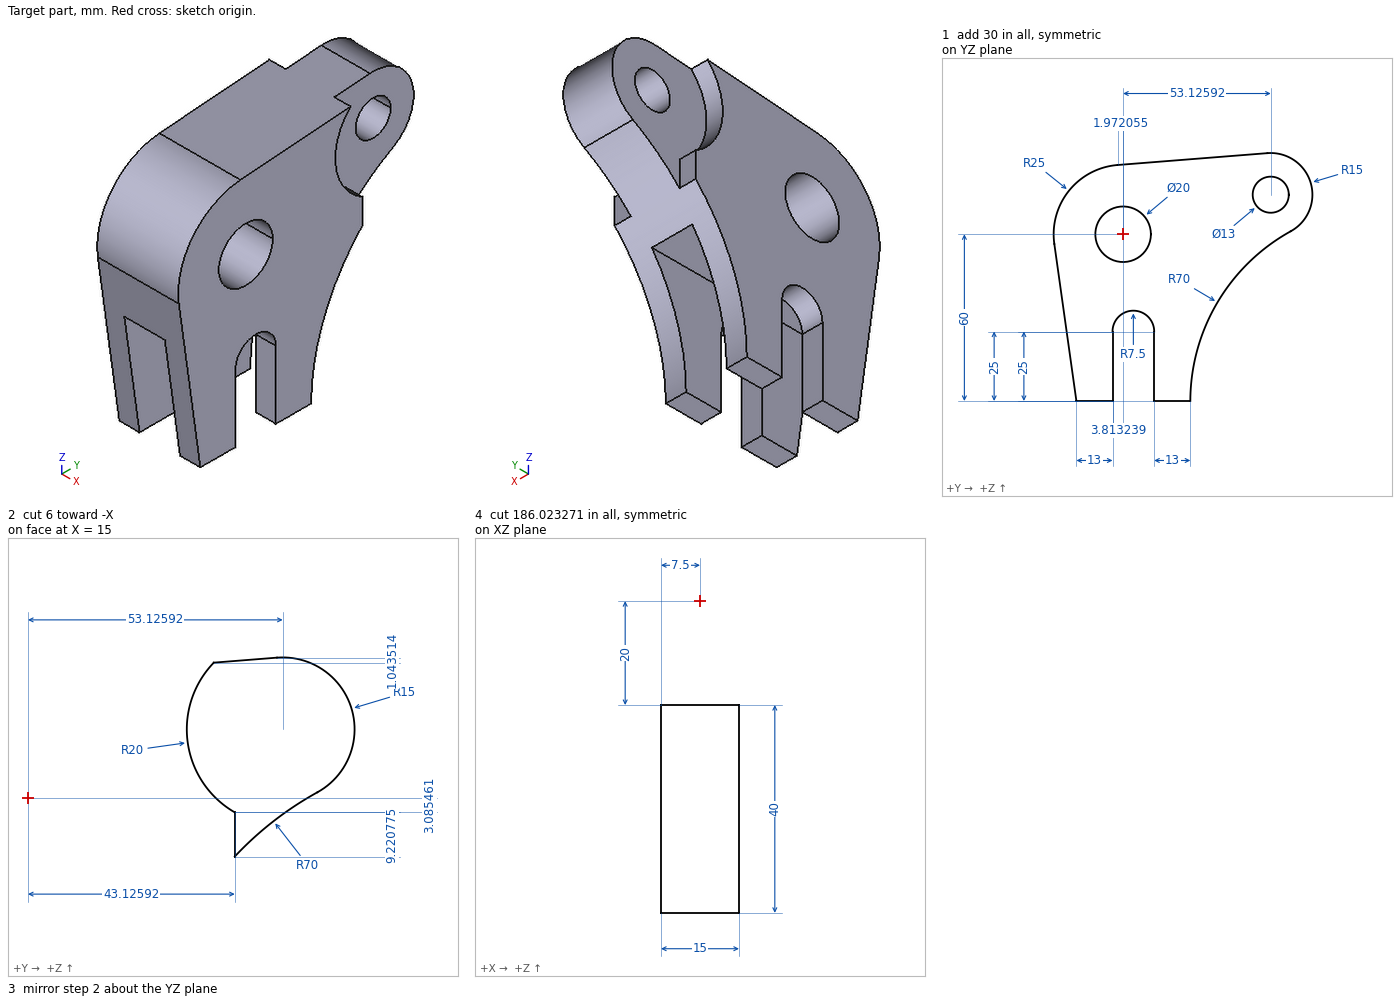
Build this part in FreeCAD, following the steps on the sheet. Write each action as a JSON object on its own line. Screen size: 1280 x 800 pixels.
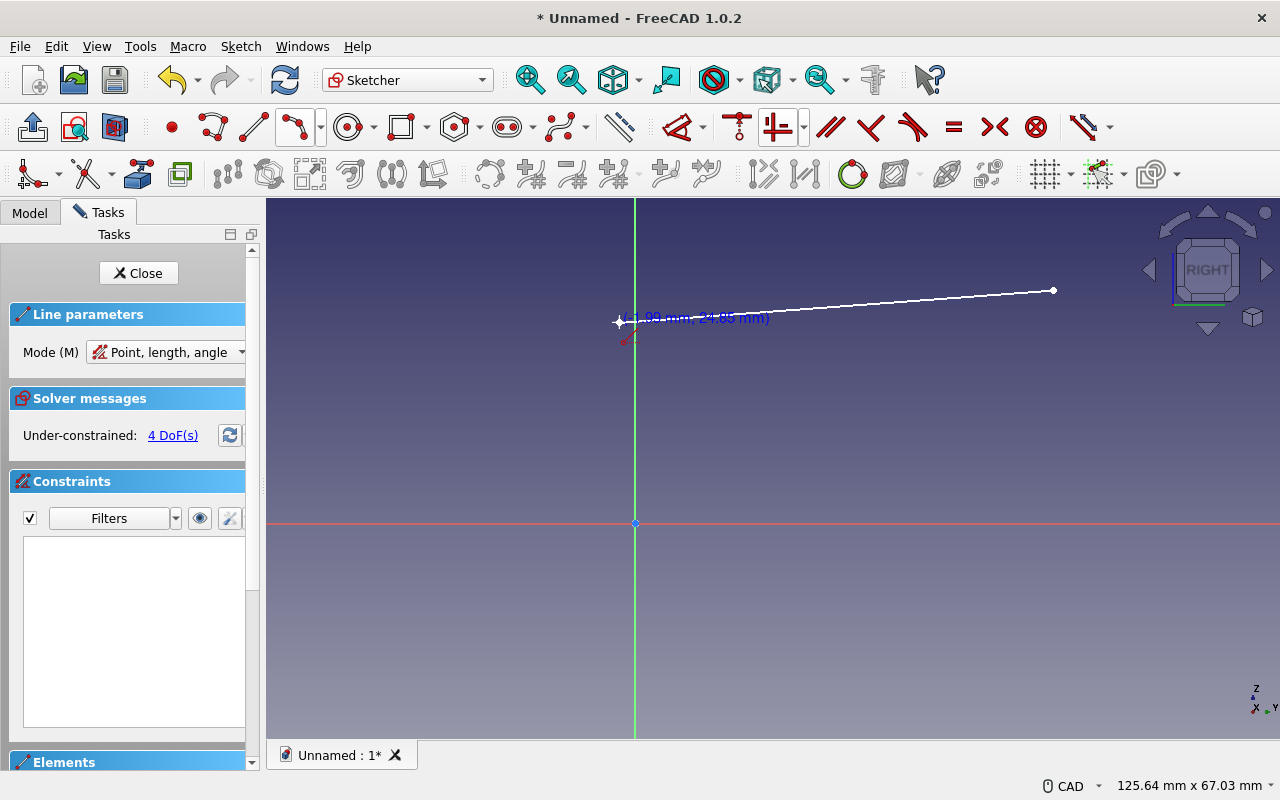
{"action": "left_click", "coordinate": [213, 128]}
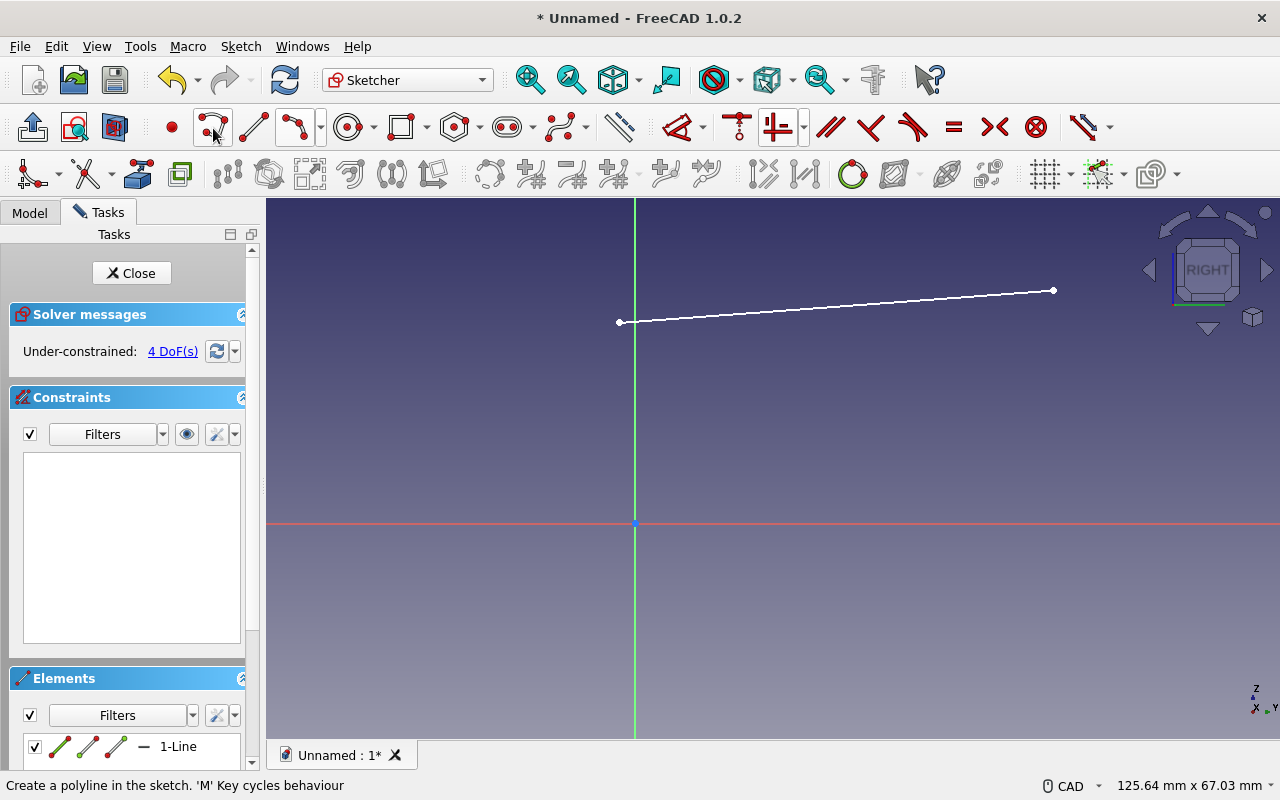
{"action": "left_click", "coordinate": [435, 552]}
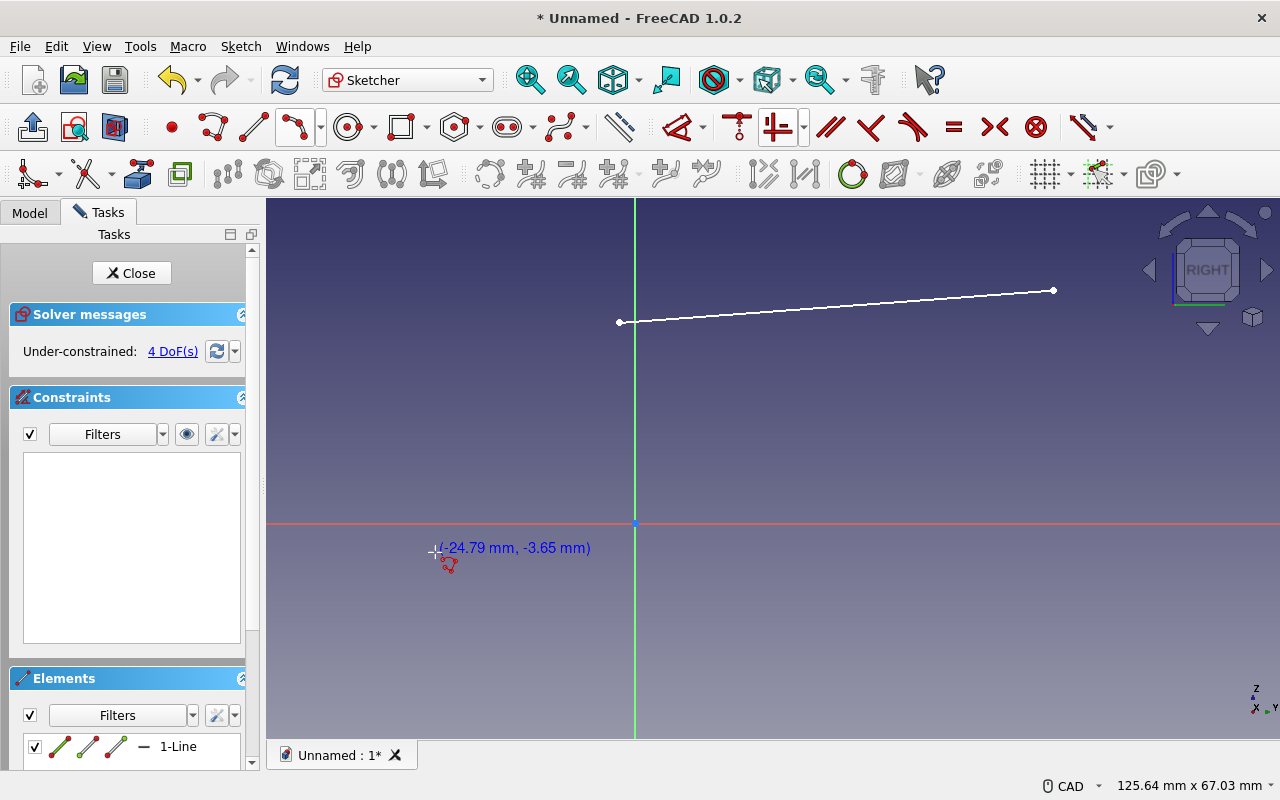
{"action": "scroll", "coordinate": [620, 322], "scroll_direction": "down", "scroll_amount": 4}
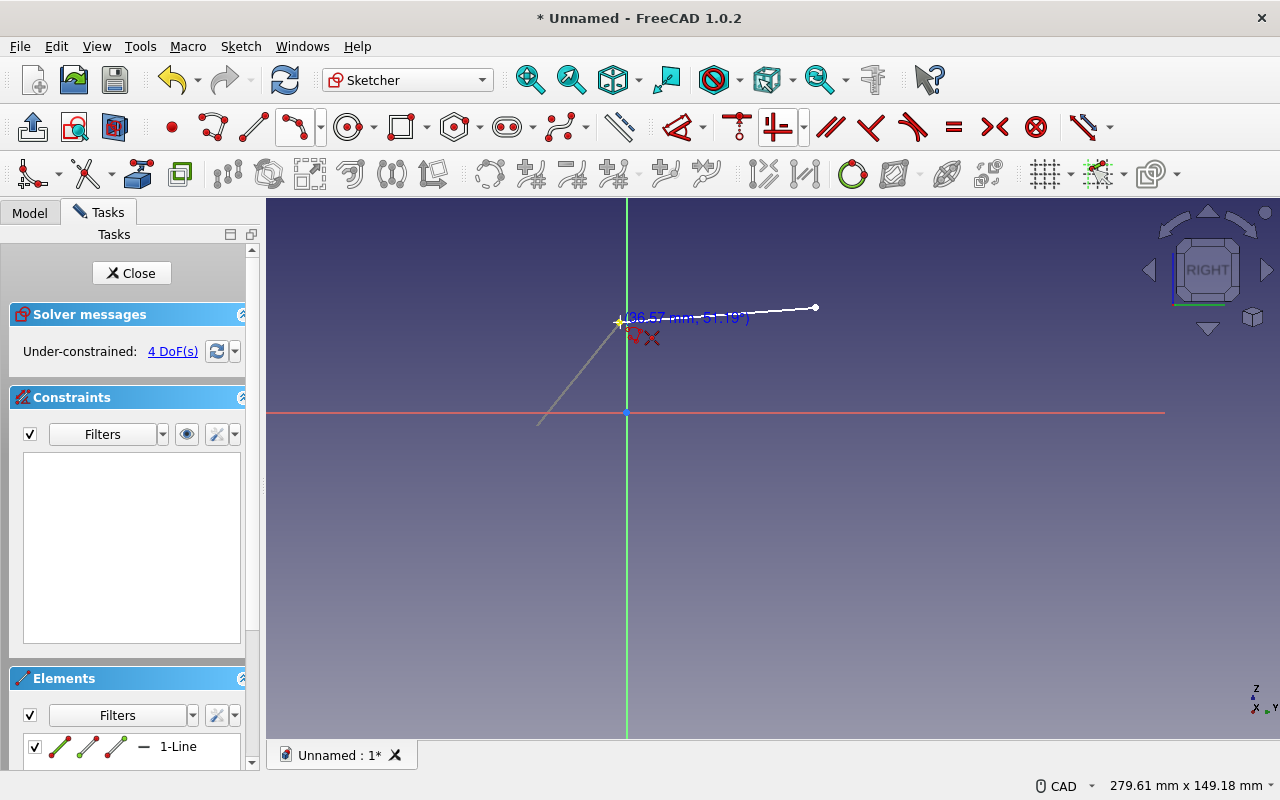
{"action": "left_click", "coordinate": [566, 630]}
{"action": "left_click", "coordinate": [613, 630]}
{"action": "left_click", "coordinate": [613, 540]}
{"action": "right_click", "coordinate": [613, 540]}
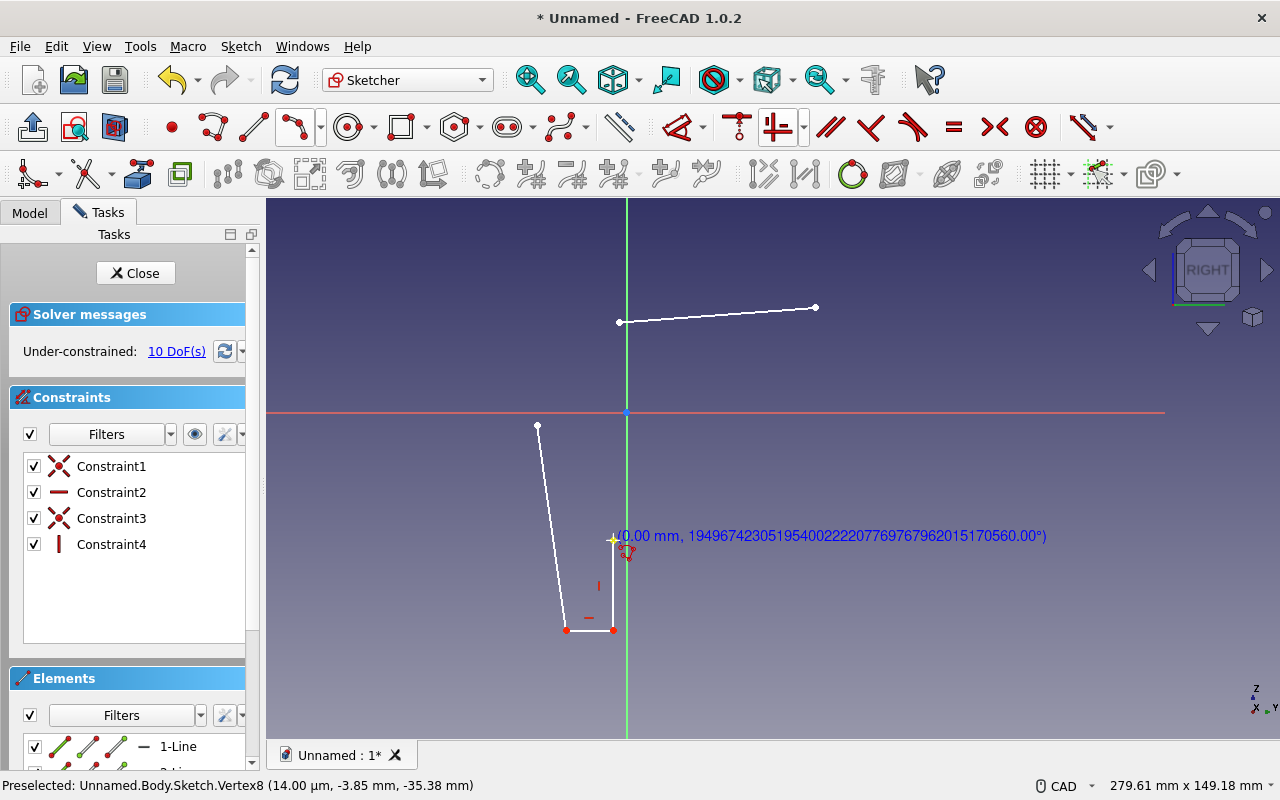
{"action": "left_click", "coordinate": [668, 540]}
{"action": "left_click", "coordinate": [668, 630]}
{"action": "left_click", "coordinate": [715, 630]}
{"action": "right_click", "coordinate": [715, 630]}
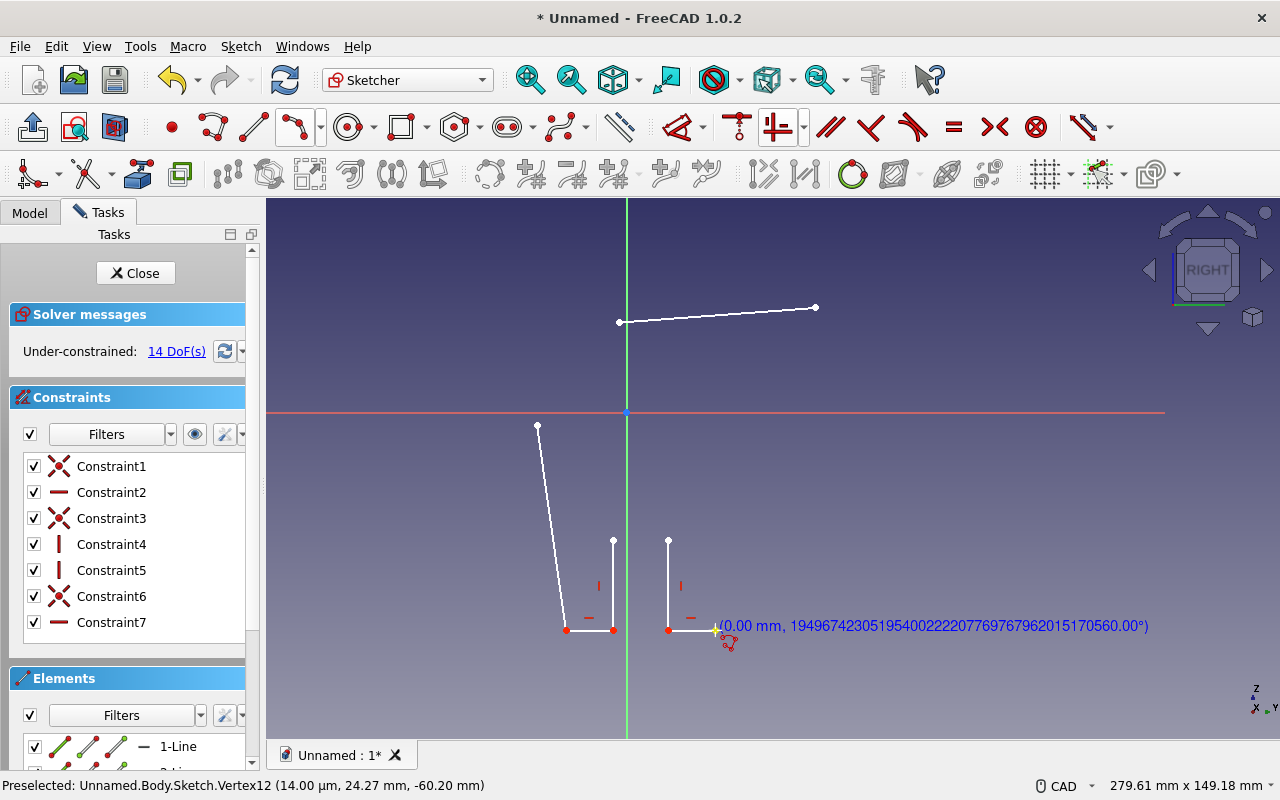
{"action": "left_click", "coordinate": [294, 128]}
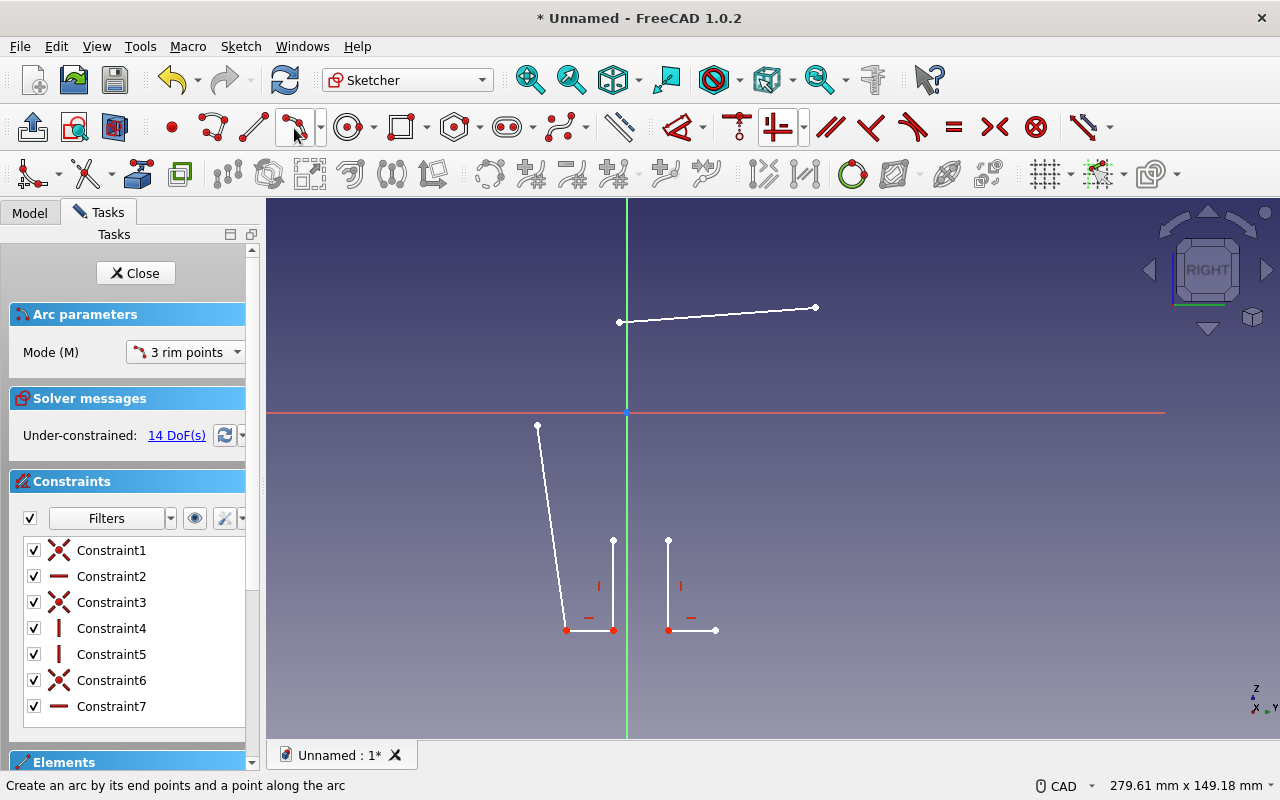
{"action": "scroll", "coordinate": [620, 322], "scroll_direction": "up", "scroll_amount": 4}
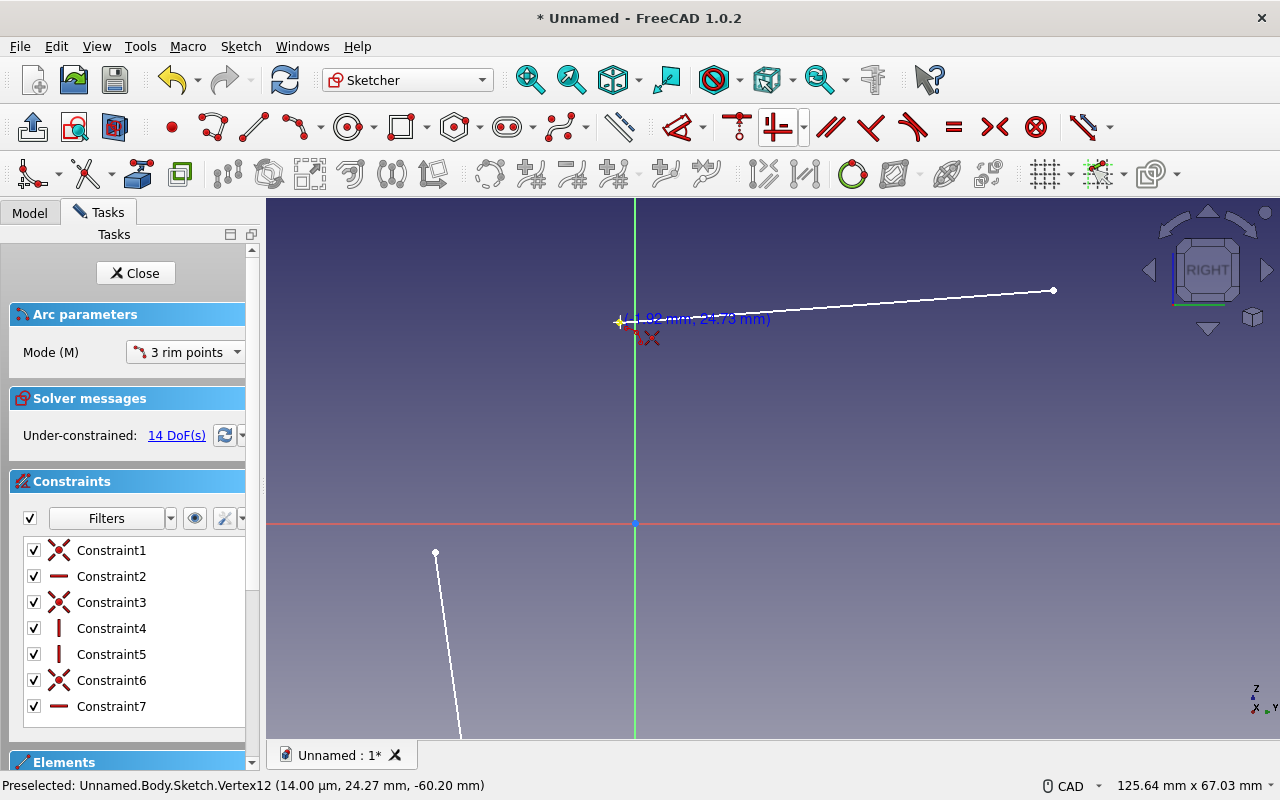
{"action": "left_click", "coordinate": [619, 323]}
{"action": "left_click", "coordinate": [435, 553]}
{"action": "left_click", "coordinate": [478, 397]}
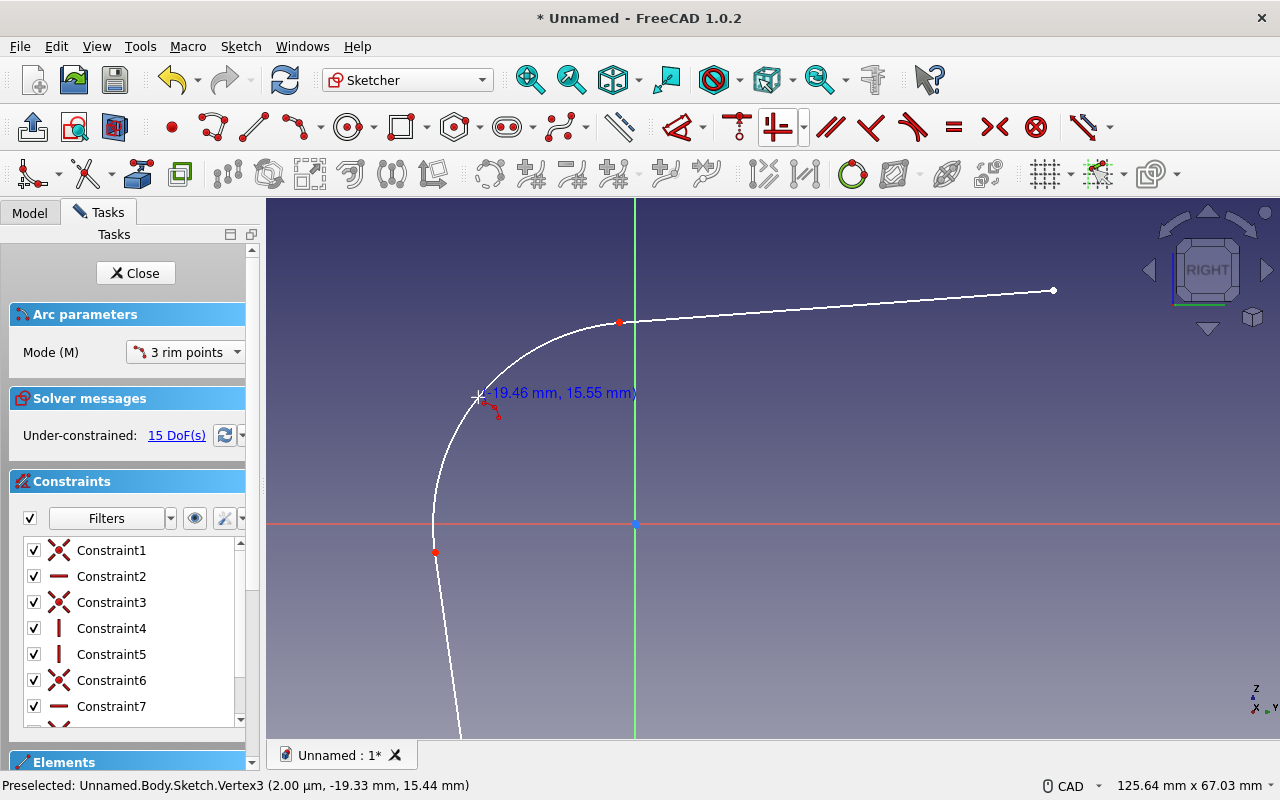
{"action": "scroll", "coordinate": [620, 322], "scroll_direction": "down", "scroll_amount": 4}